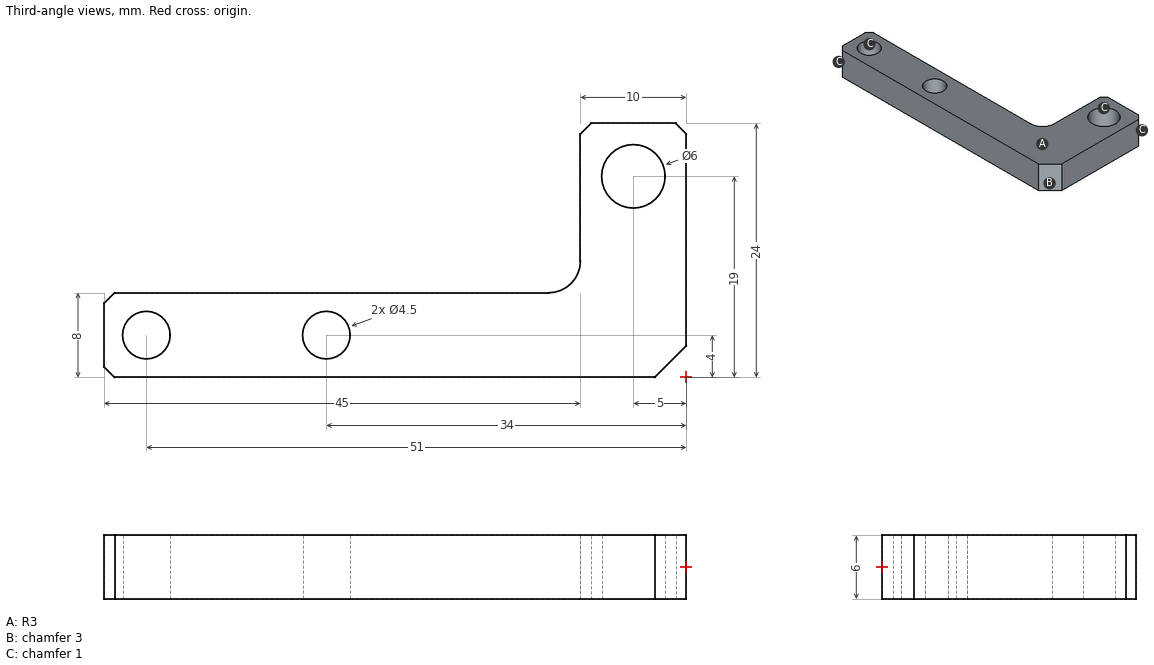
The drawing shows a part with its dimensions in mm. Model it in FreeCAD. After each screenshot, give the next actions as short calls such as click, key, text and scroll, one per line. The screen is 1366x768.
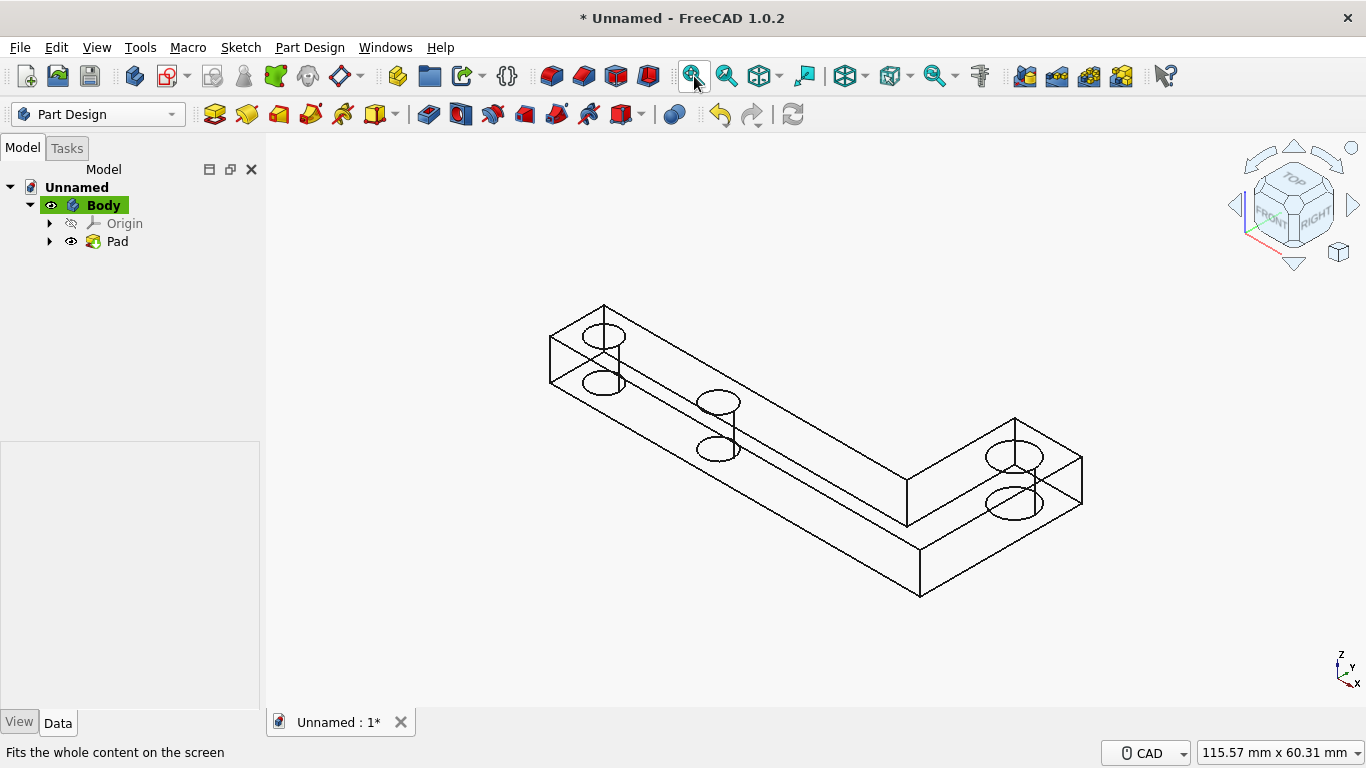
click(907, 503)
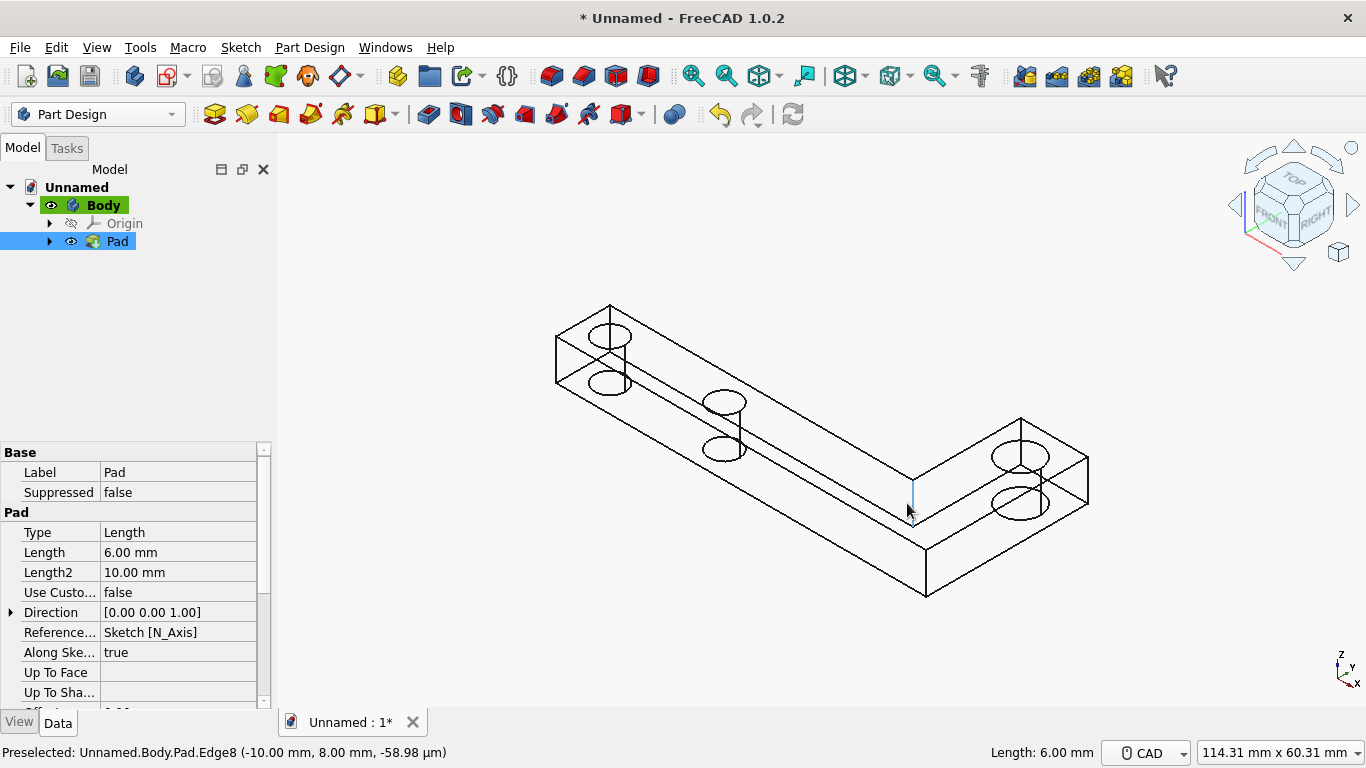
key(v)
key(1)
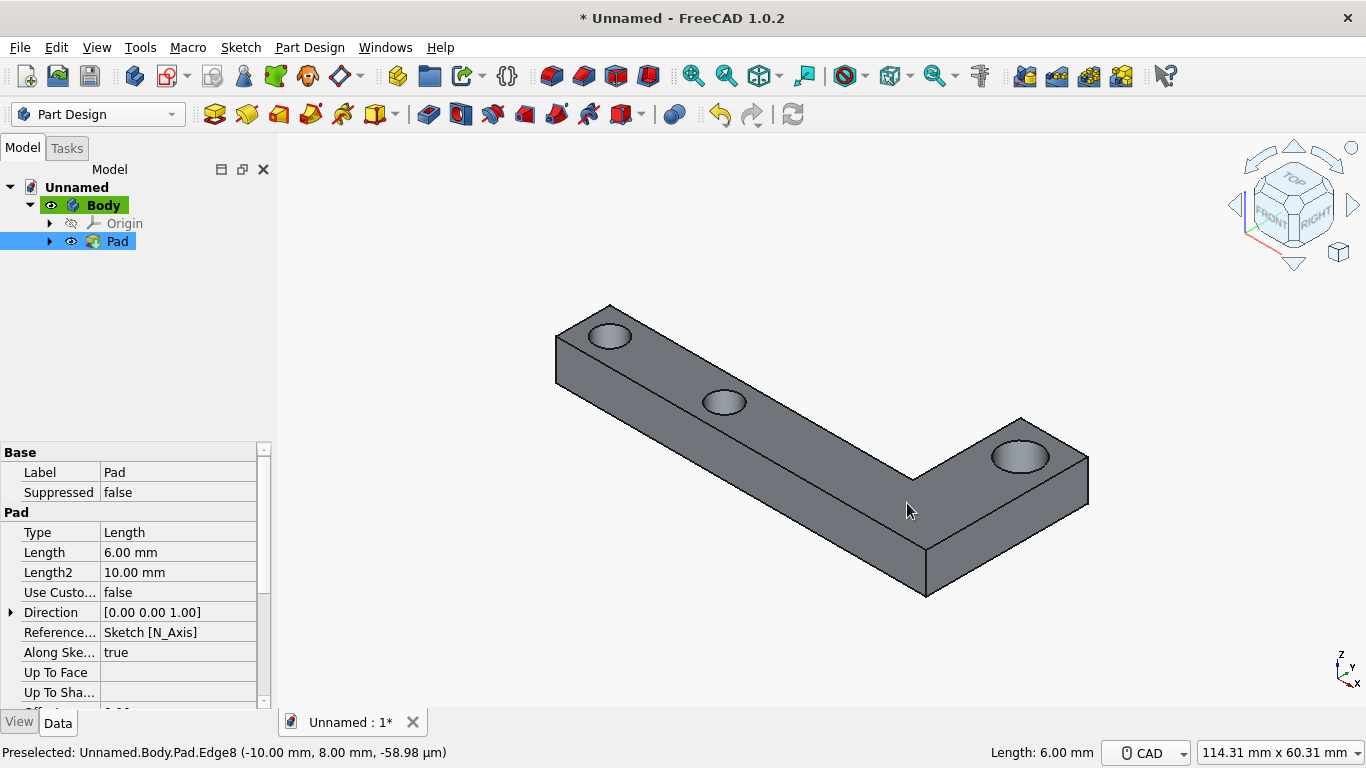
click(552, 76)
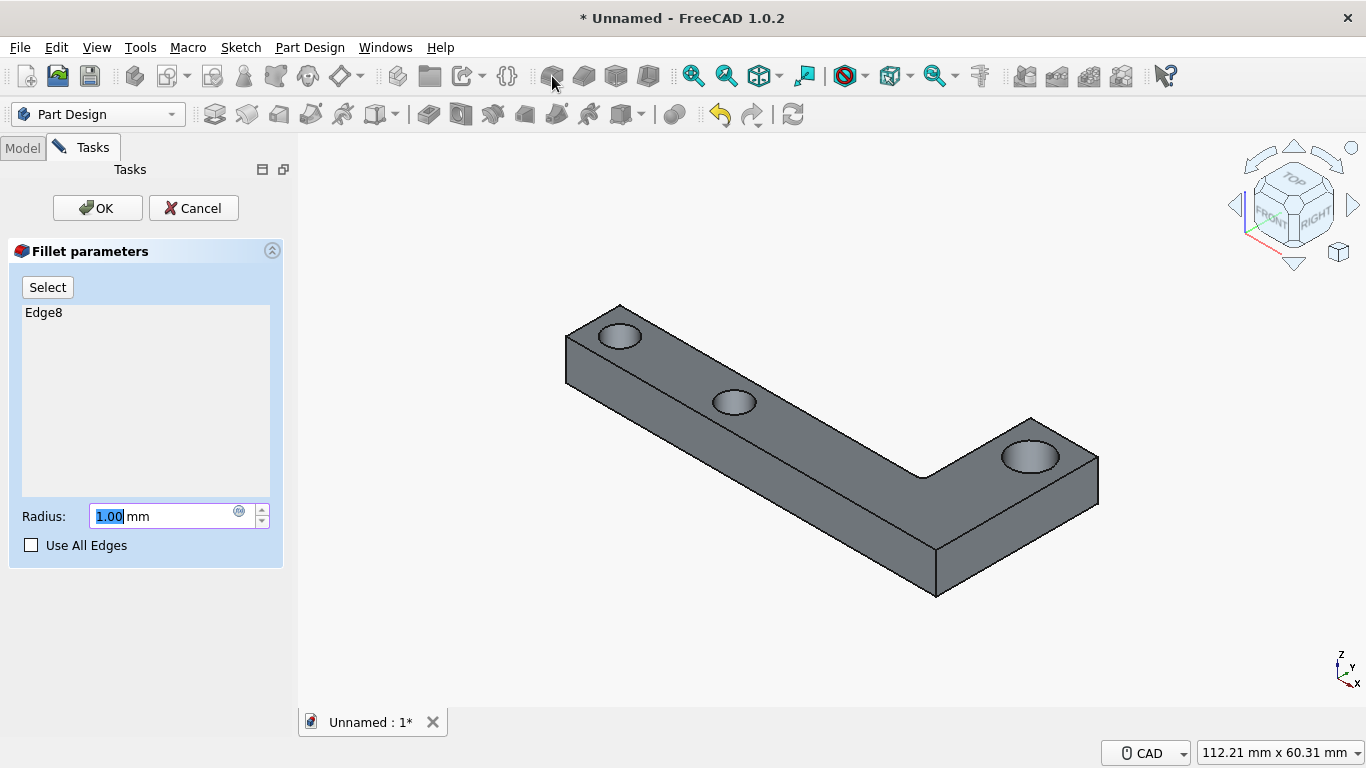
text(3)
key(Tab)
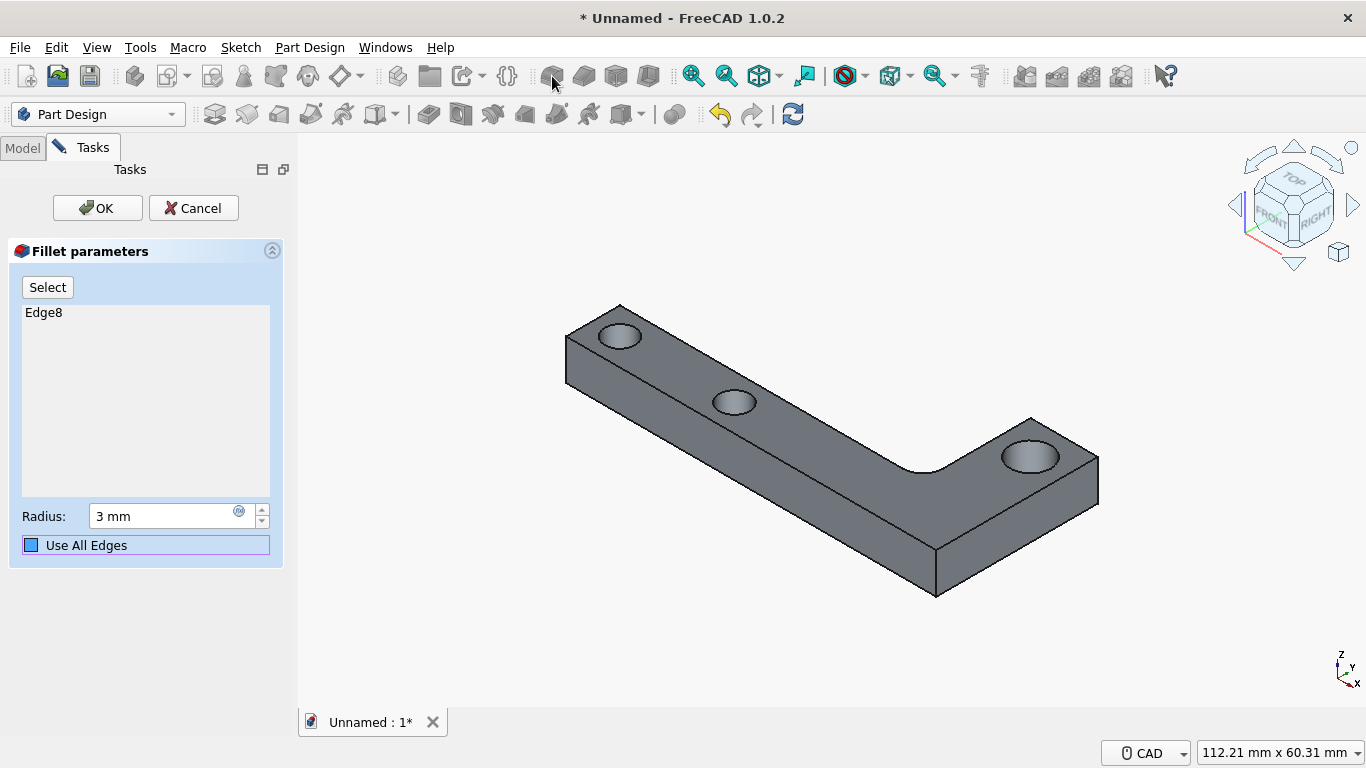
click(98, 208)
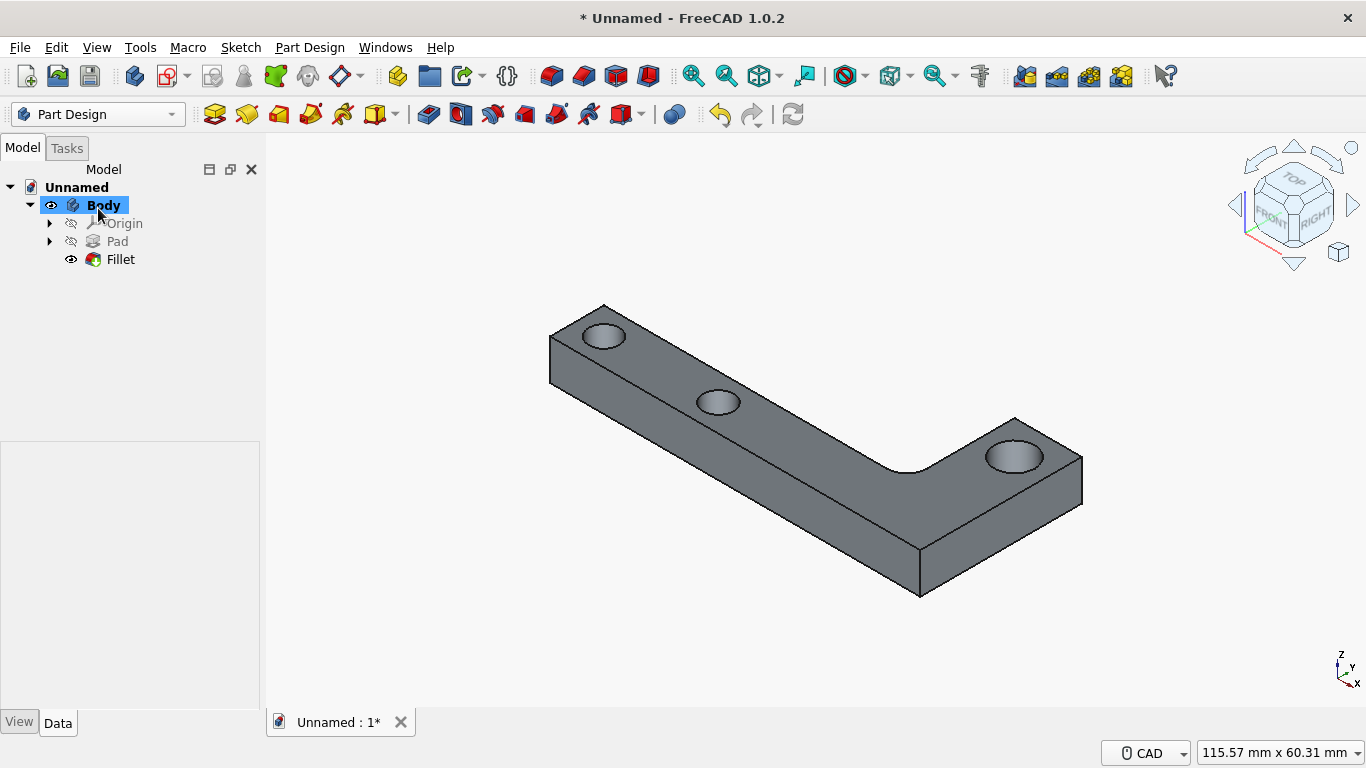
click(920, 572)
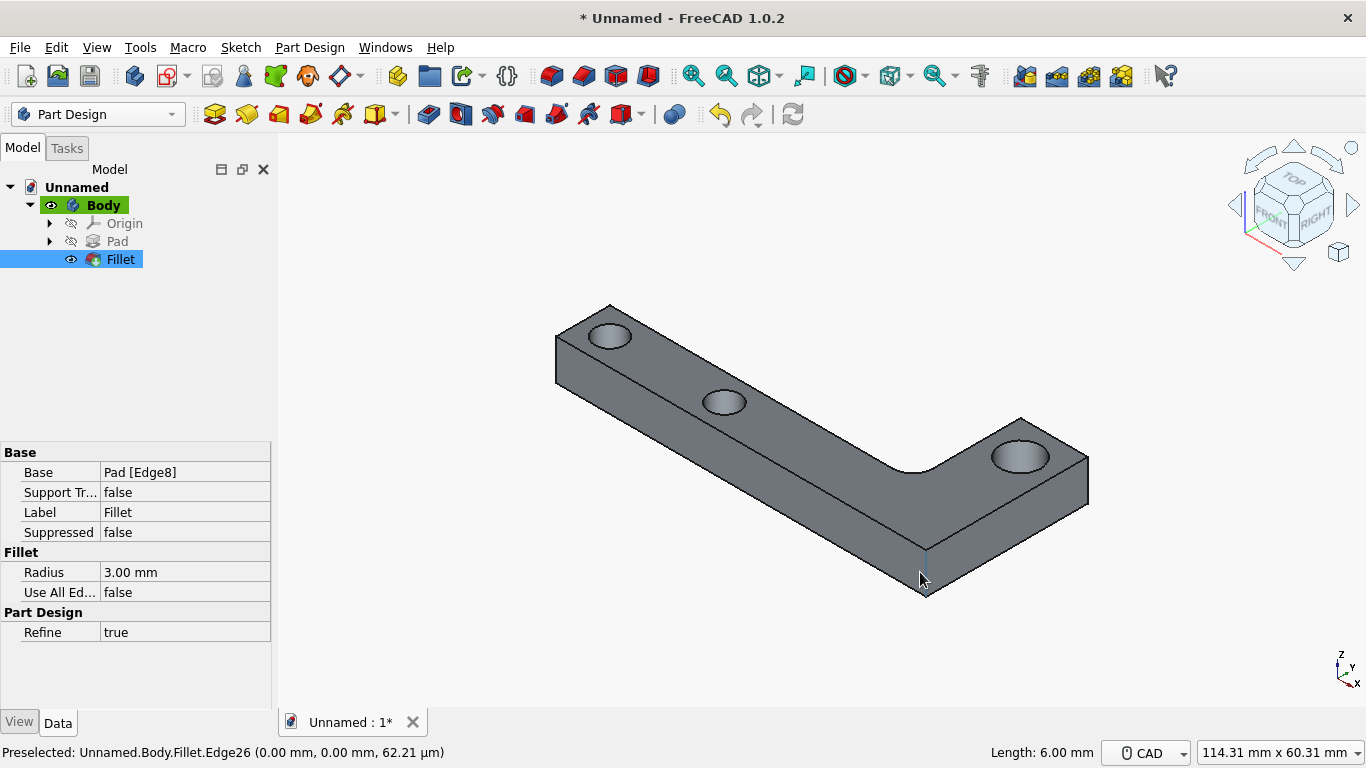
click(584, 76)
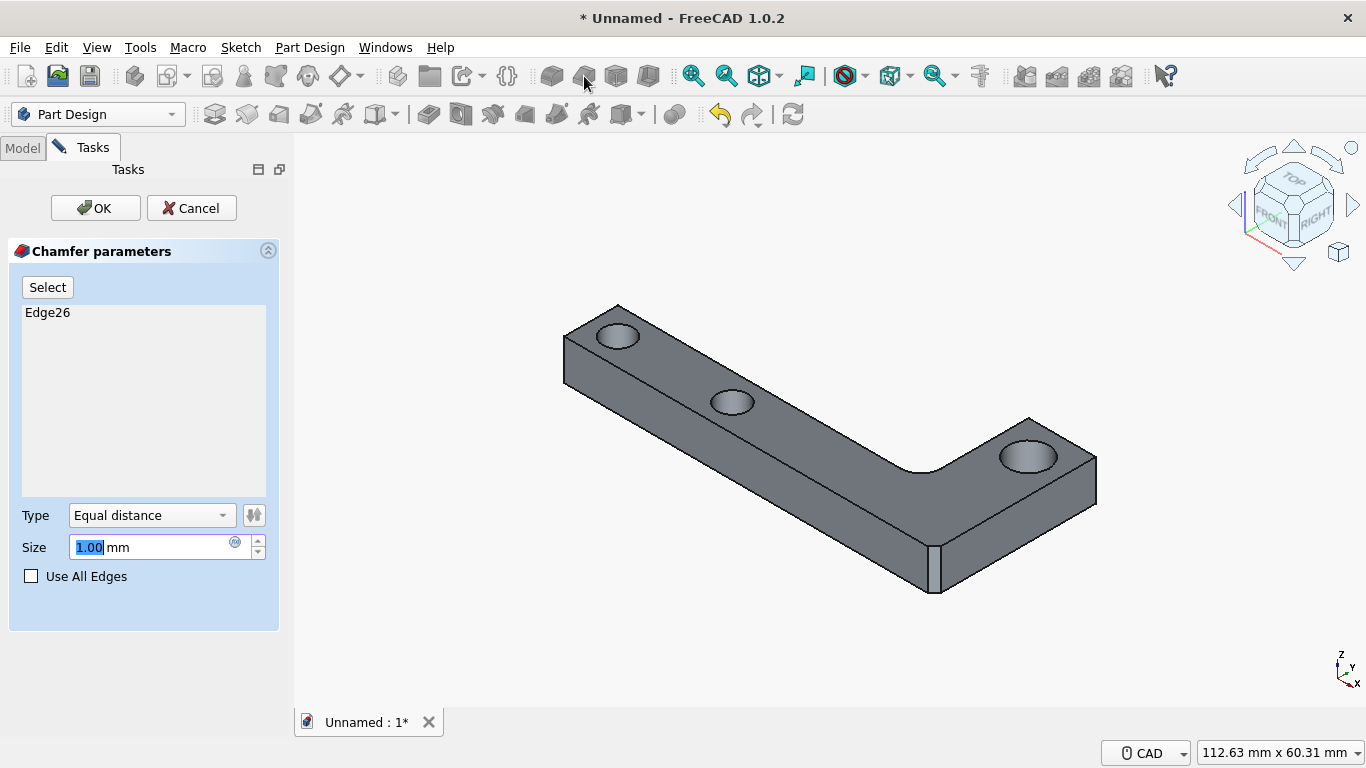
text(3)
key(Tab)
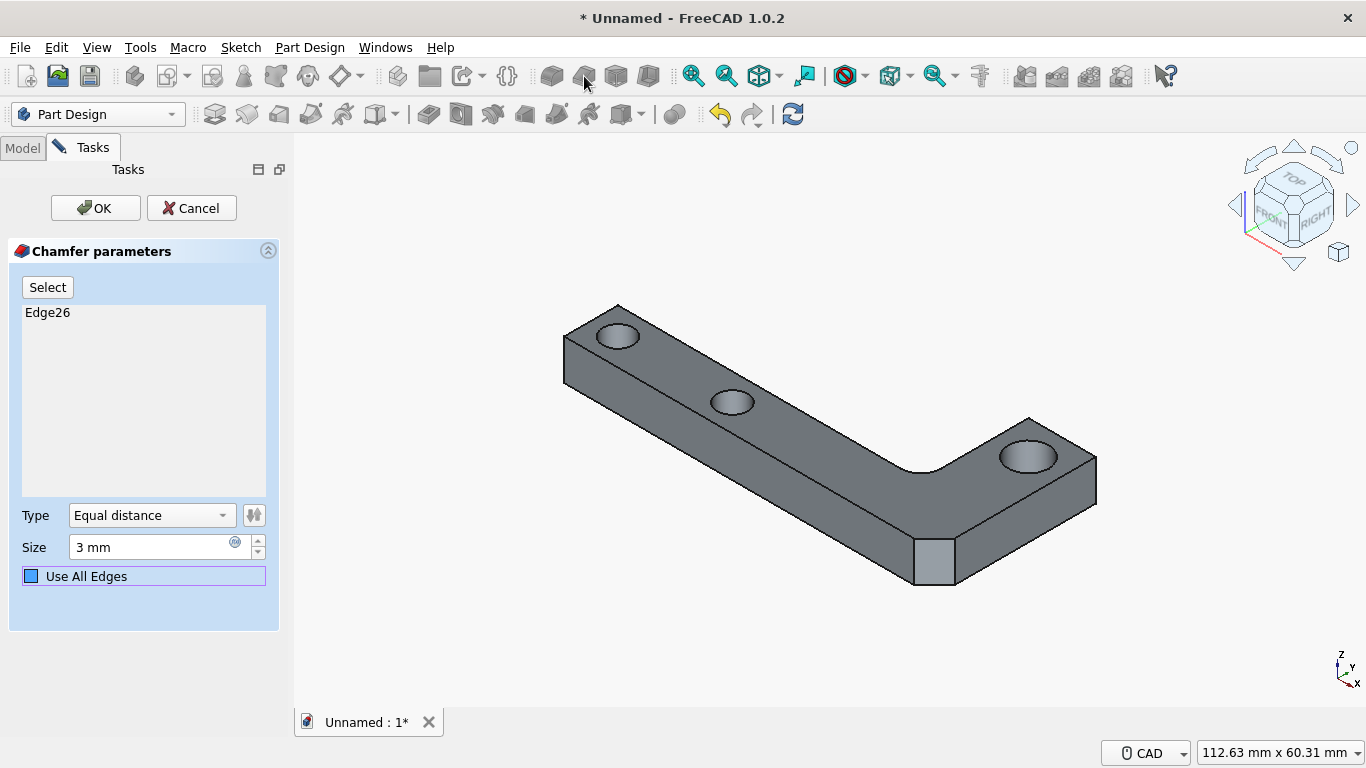
click(96, 208)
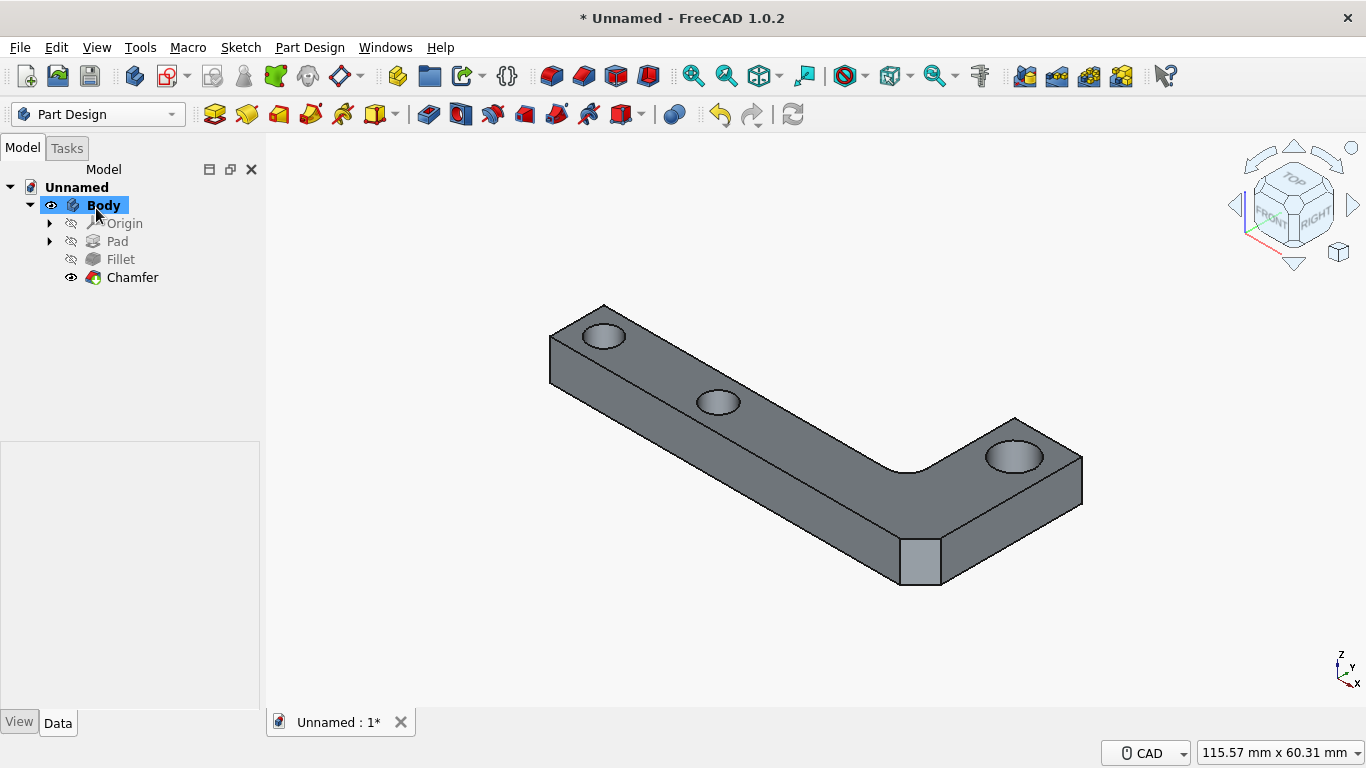
key(2)